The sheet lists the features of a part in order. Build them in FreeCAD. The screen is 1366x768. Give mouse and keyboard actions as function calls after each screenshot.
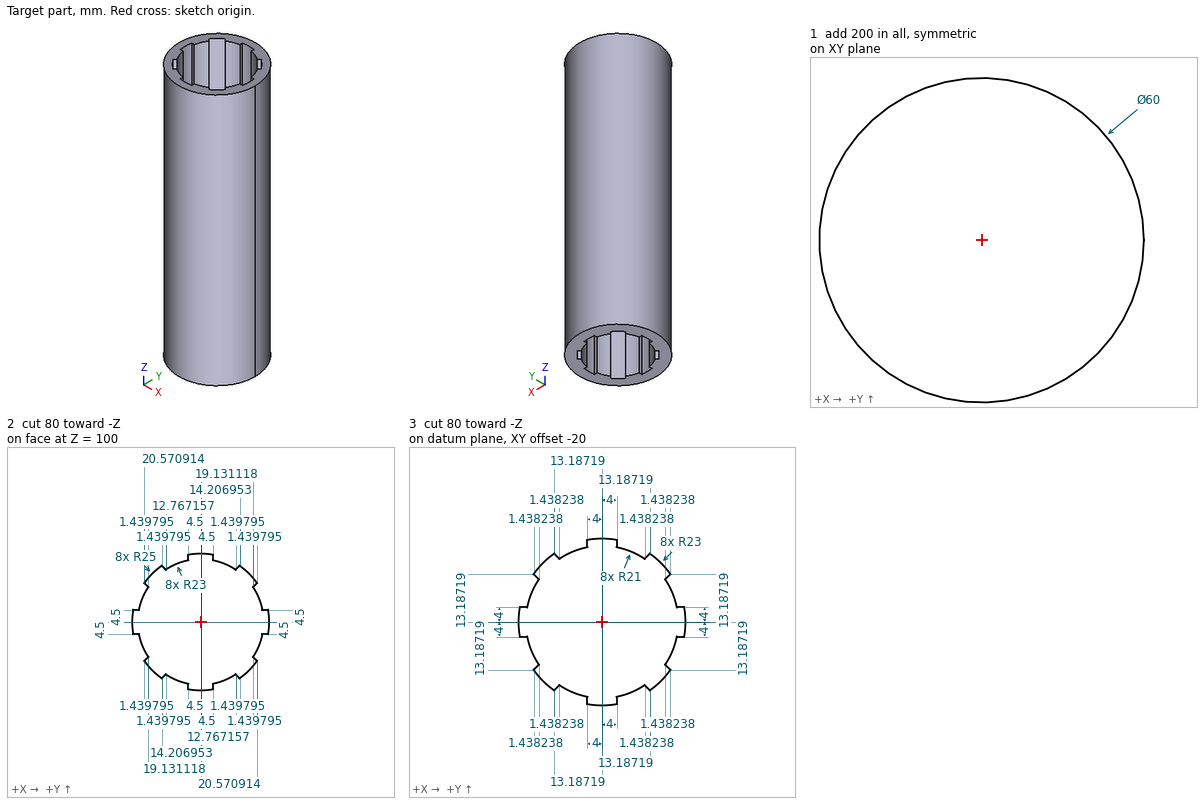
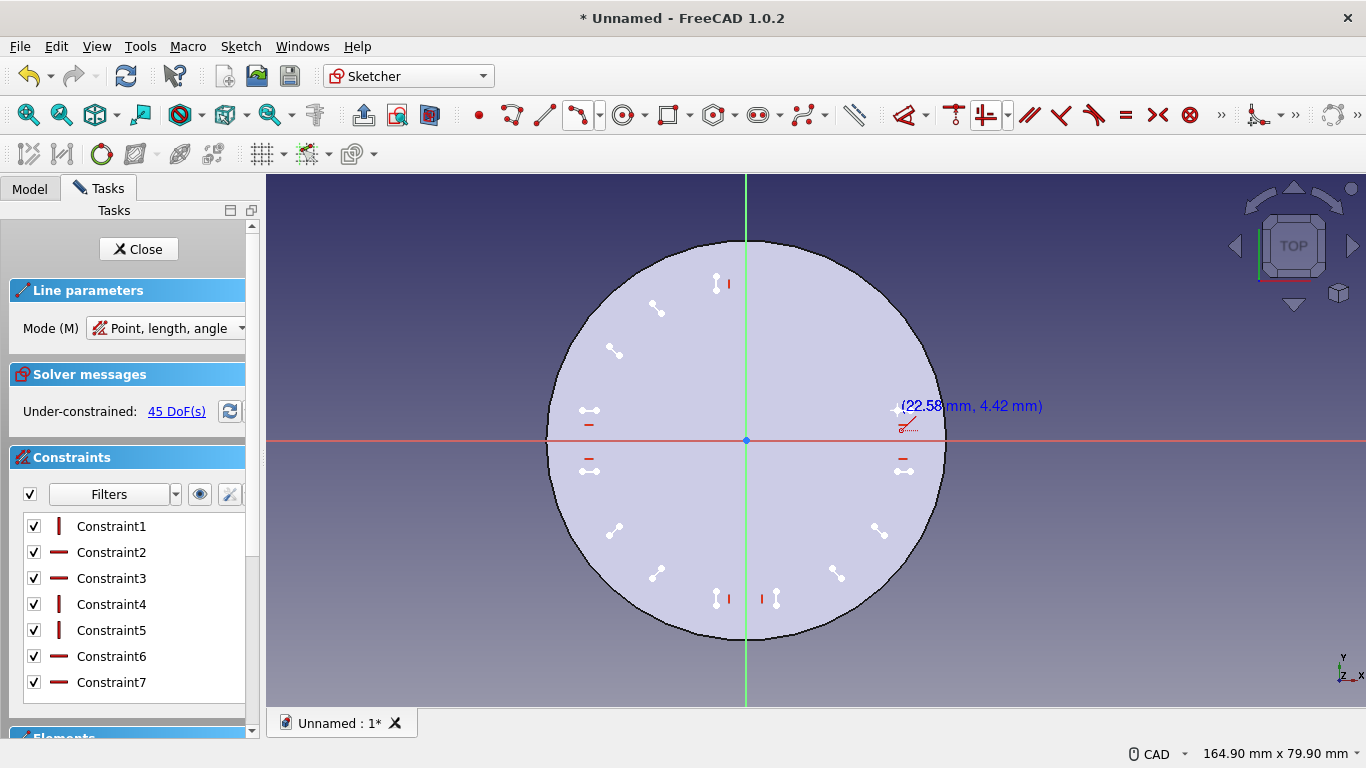
click(874, 355)
click(884, 346)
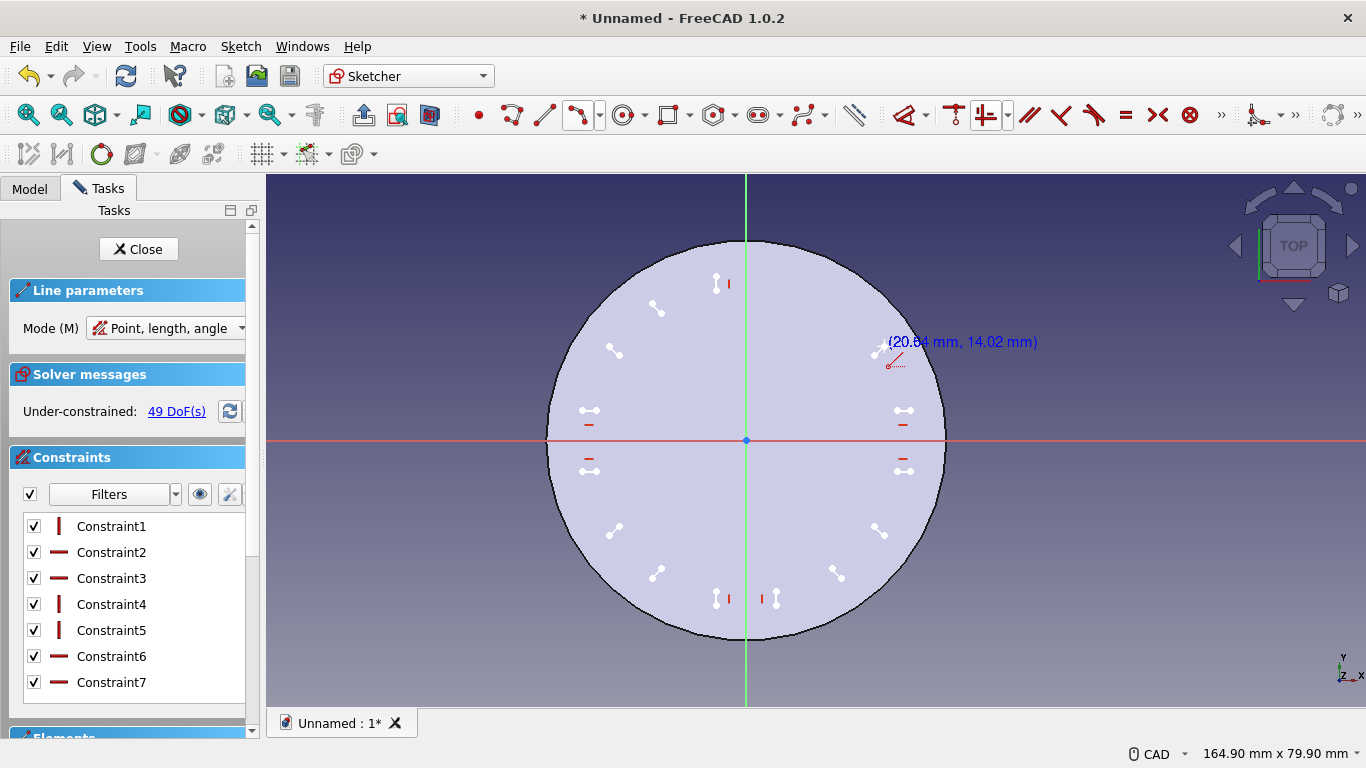
click(841, 303)
click(832, 313)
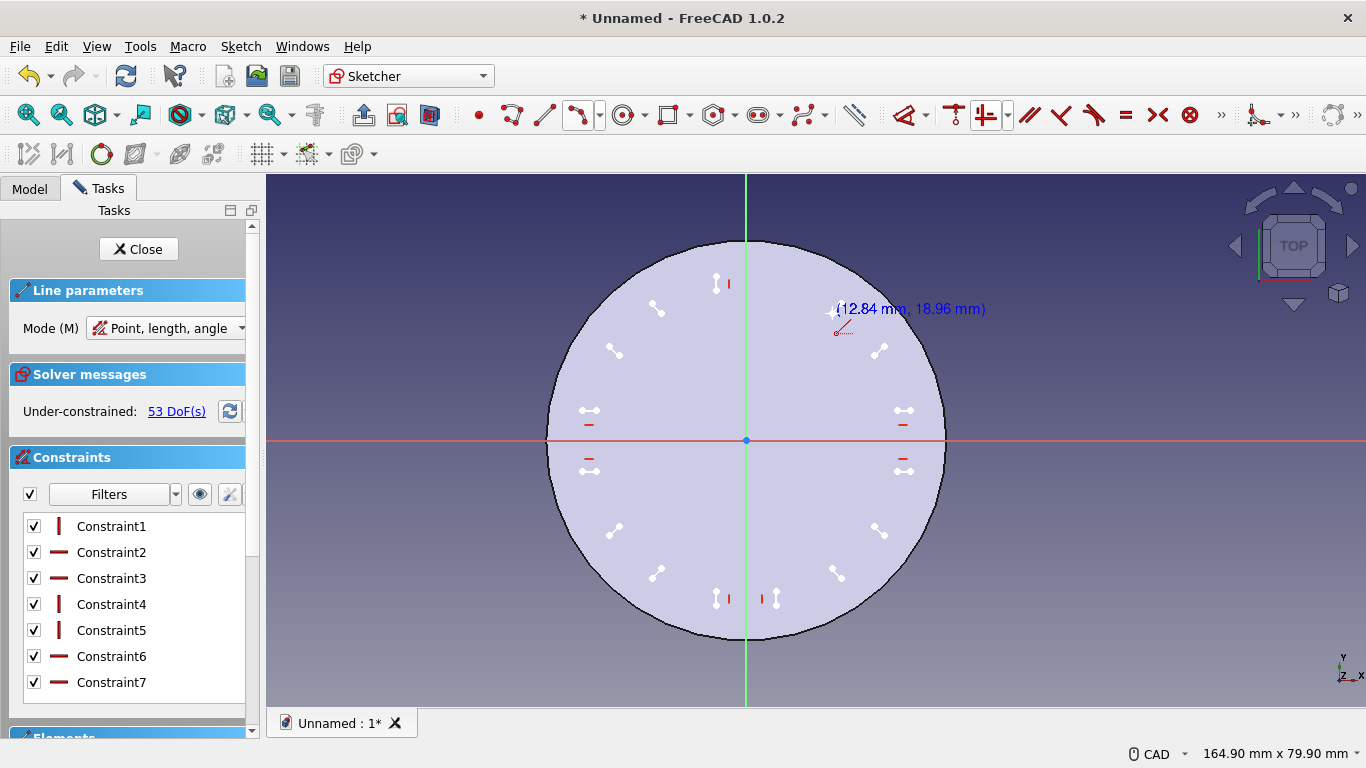
click(776, 290)
click(776, 276)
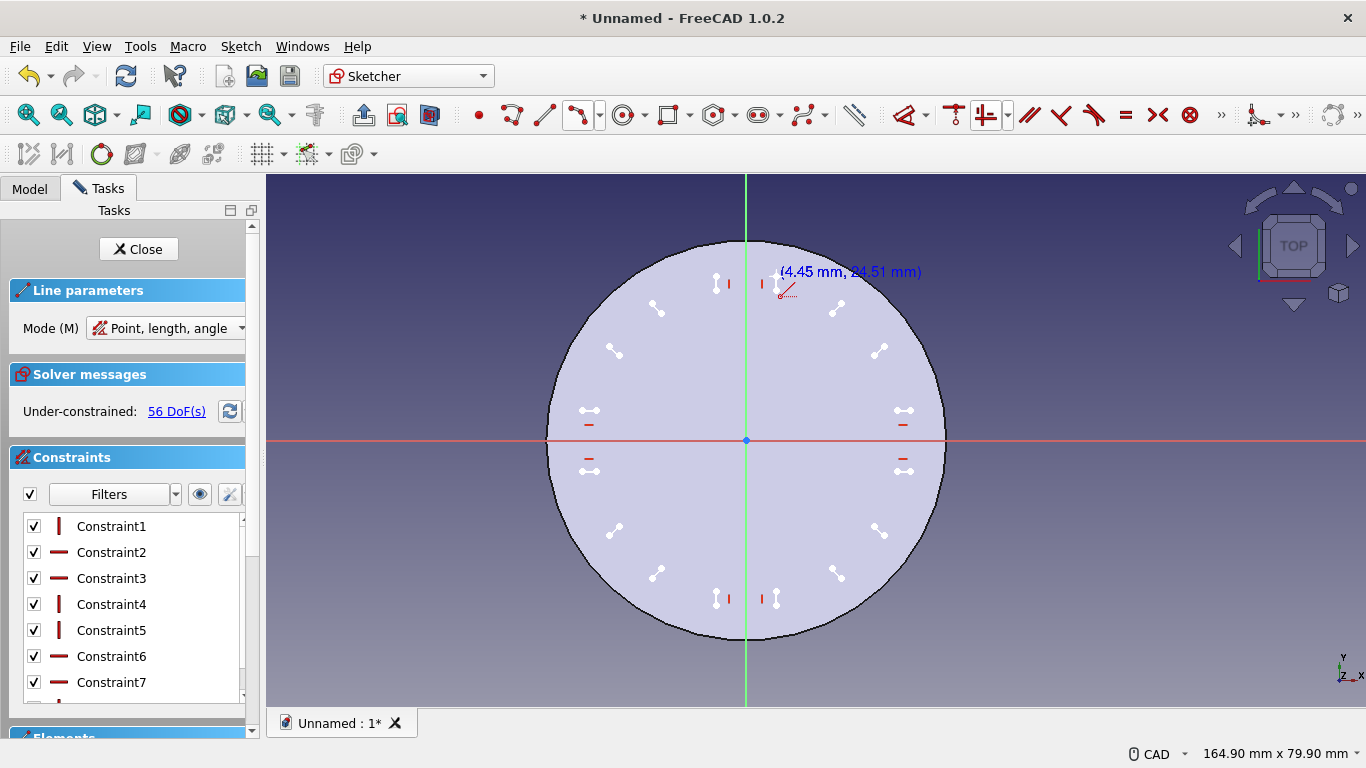
click(578, 116)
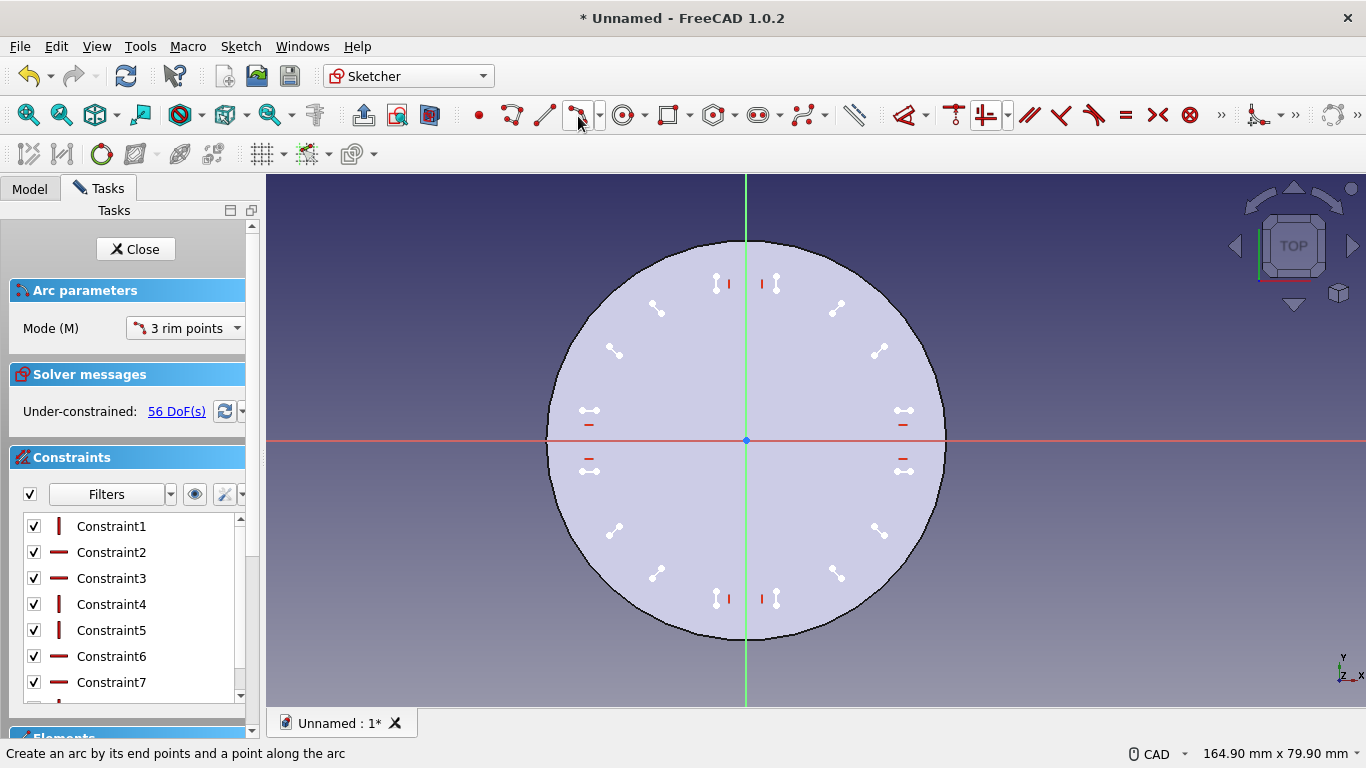
scroll(716, 290, up, 5)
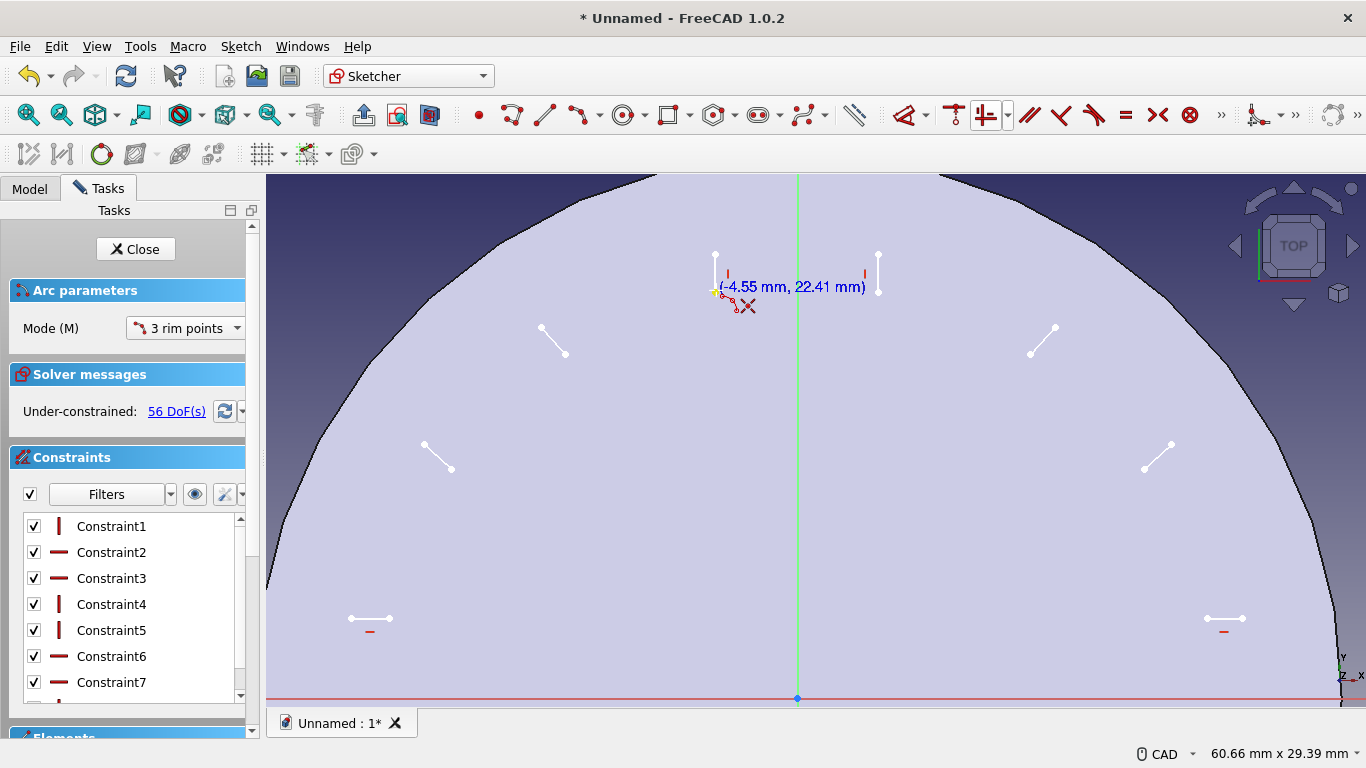
click(715, 292)
click(566, 355)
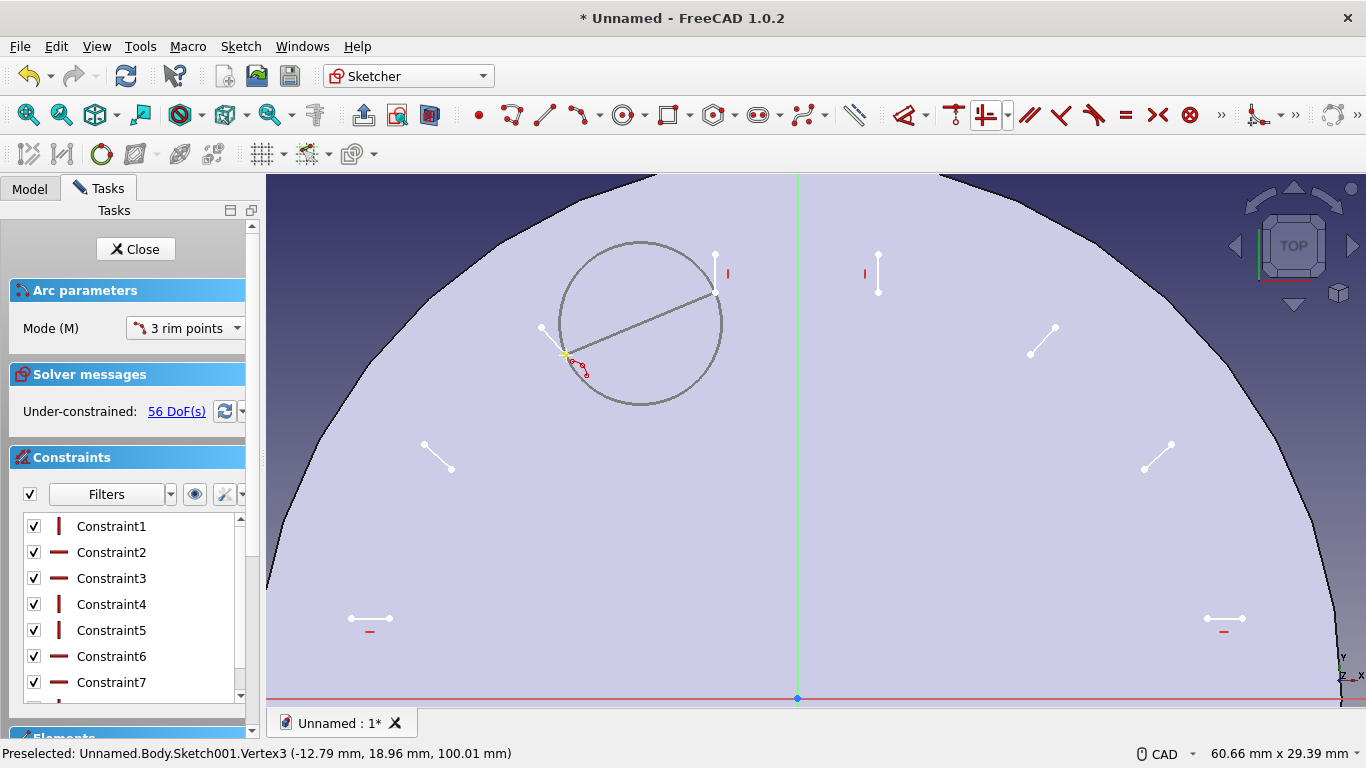
scroll(638, 313, up, 4)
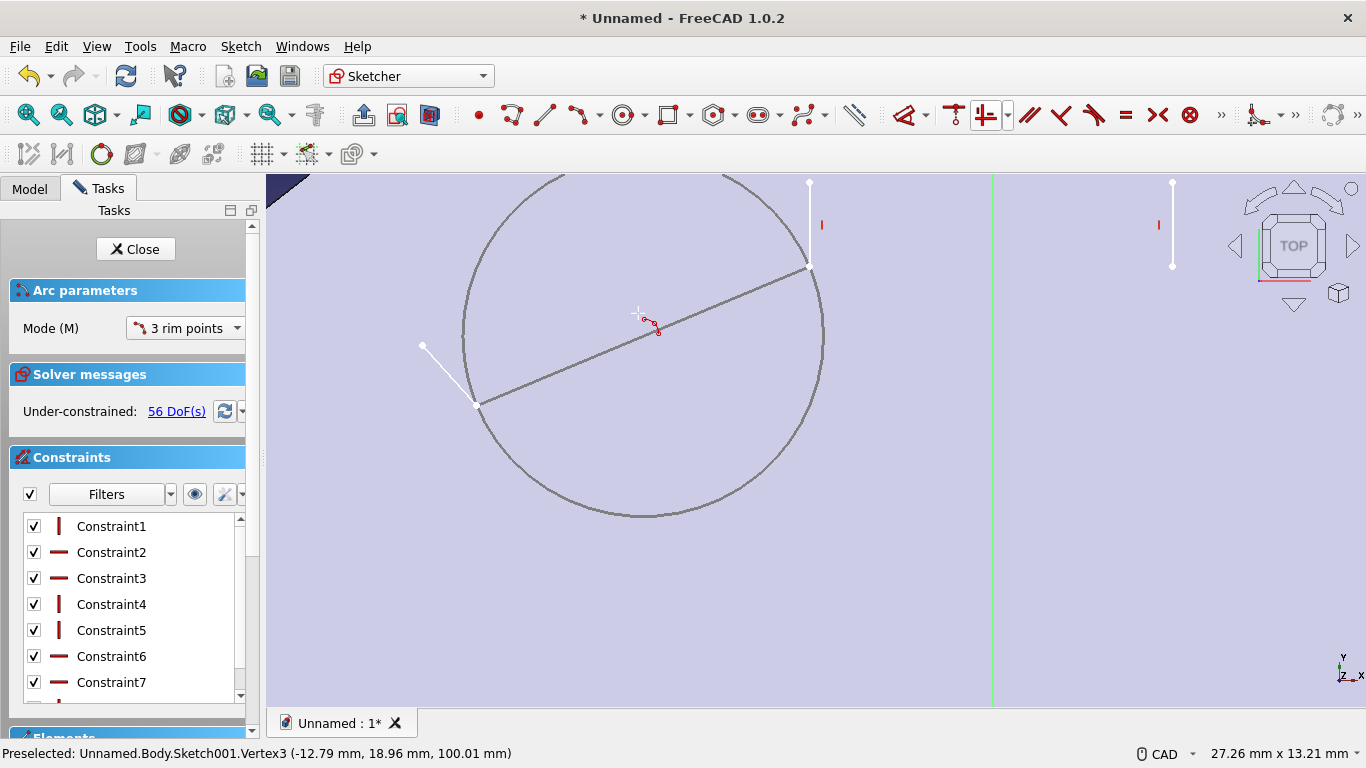
click(638, 314)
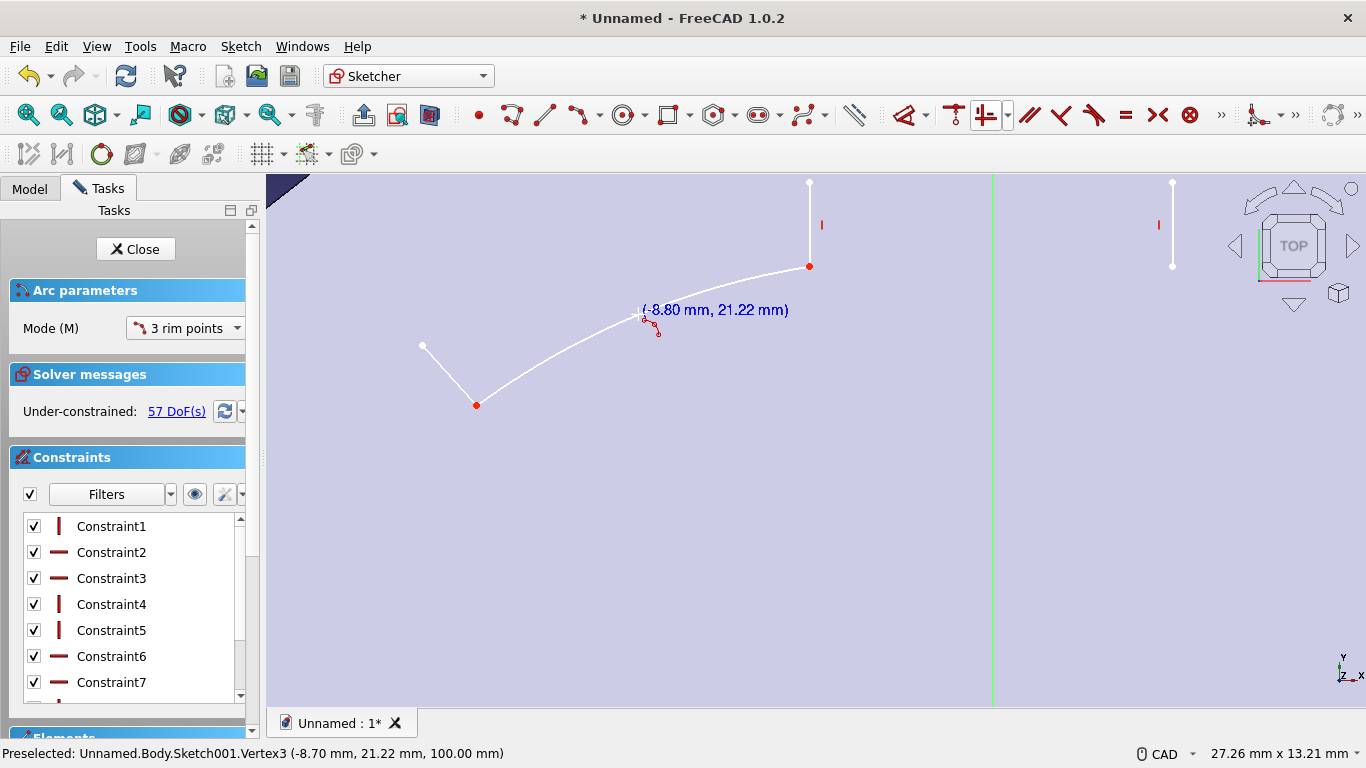
click(422, 345)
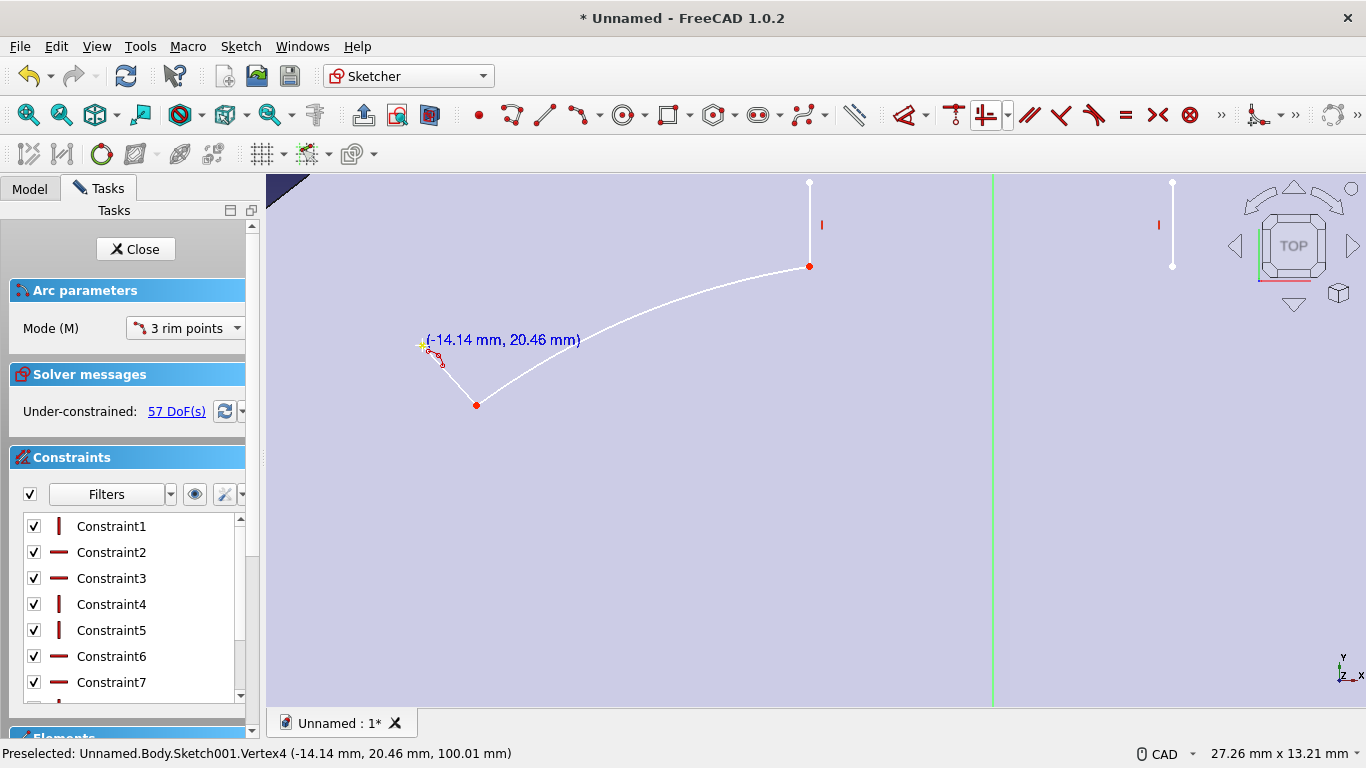
scroll(699, 296, down, 9)